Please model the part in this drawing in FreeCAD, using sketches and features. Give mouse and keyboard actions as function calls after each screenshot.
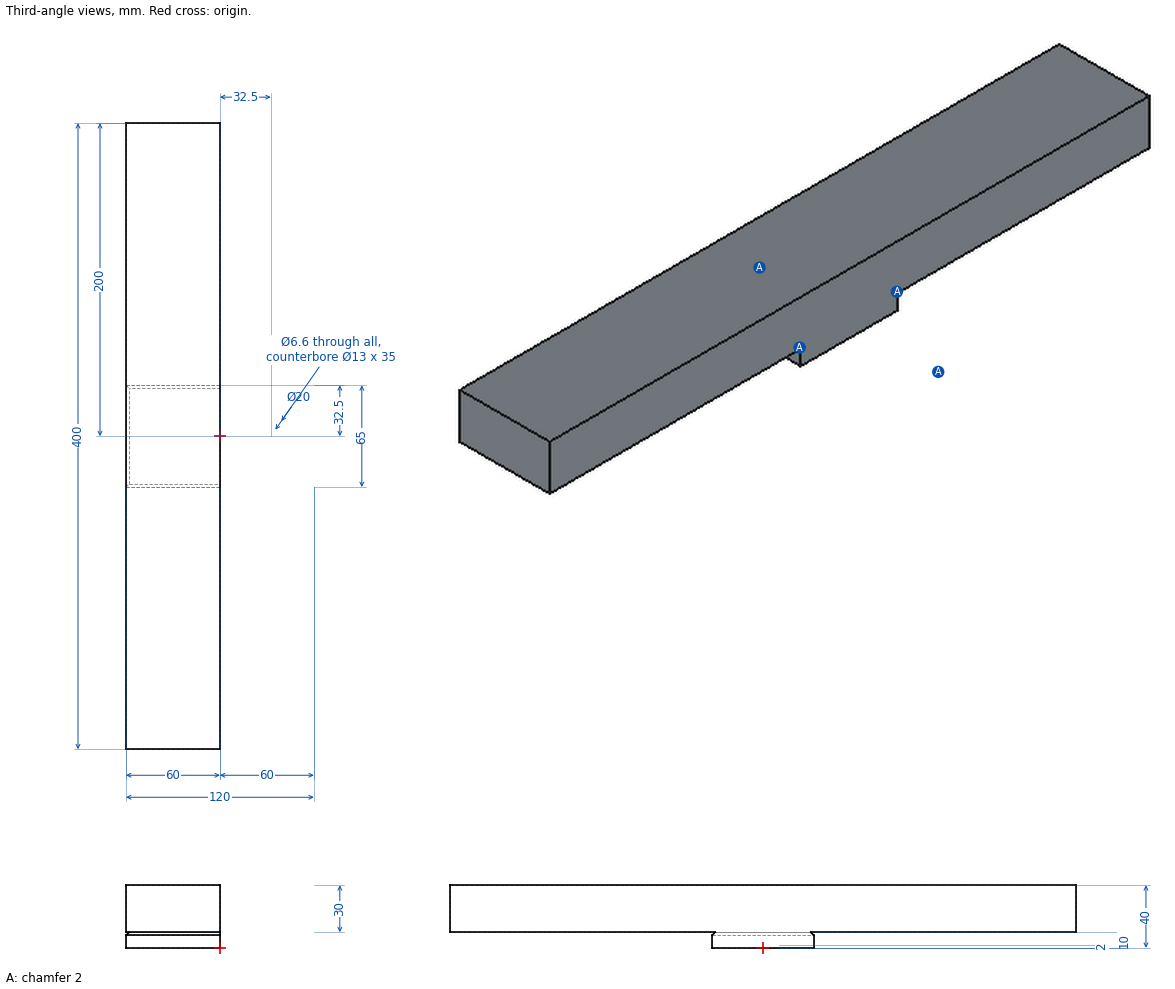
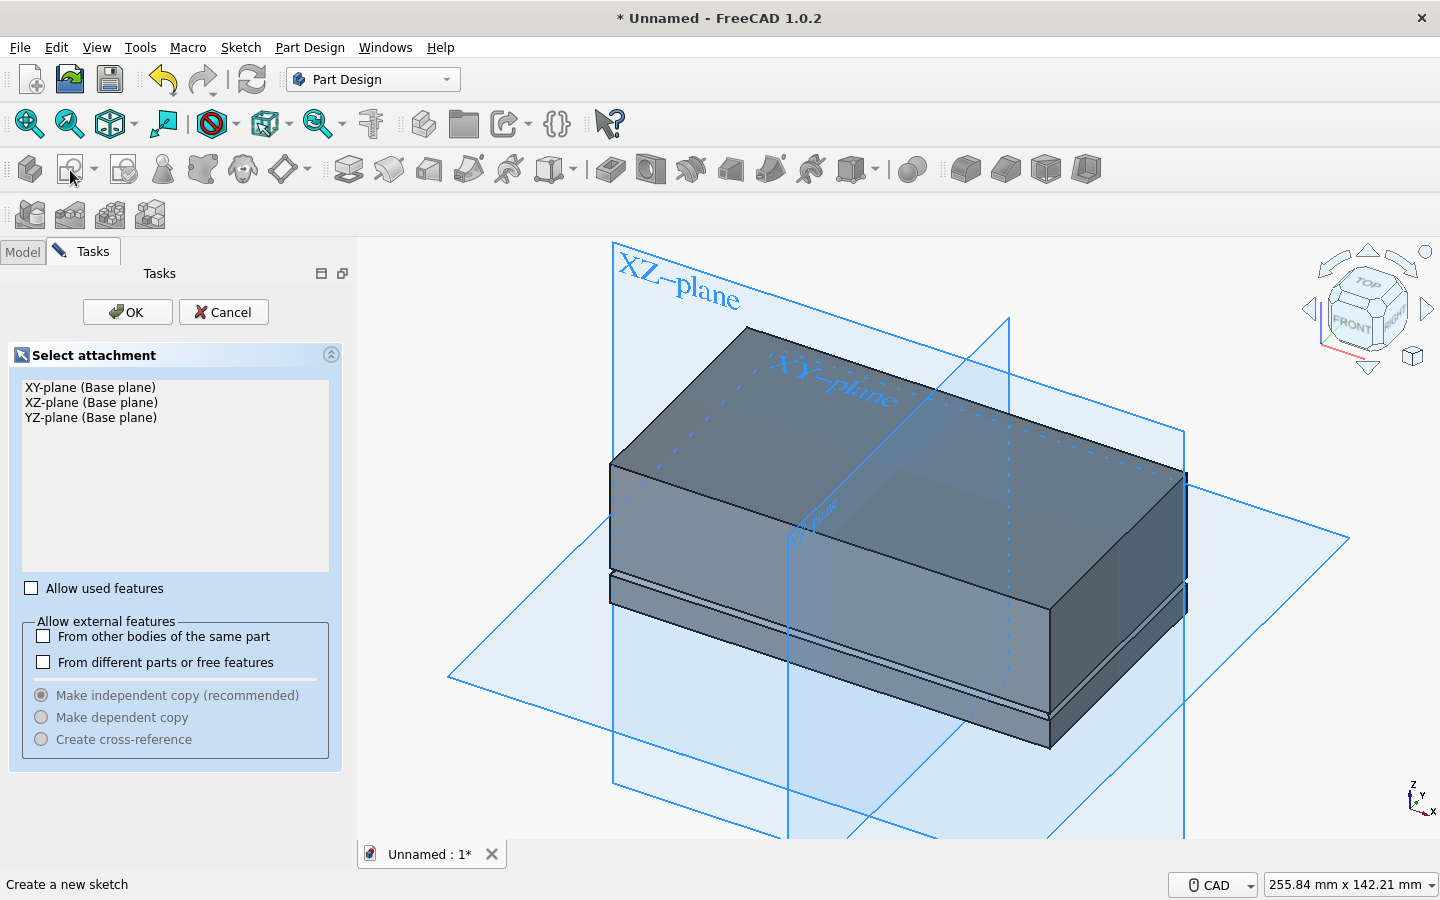
click(82, 388)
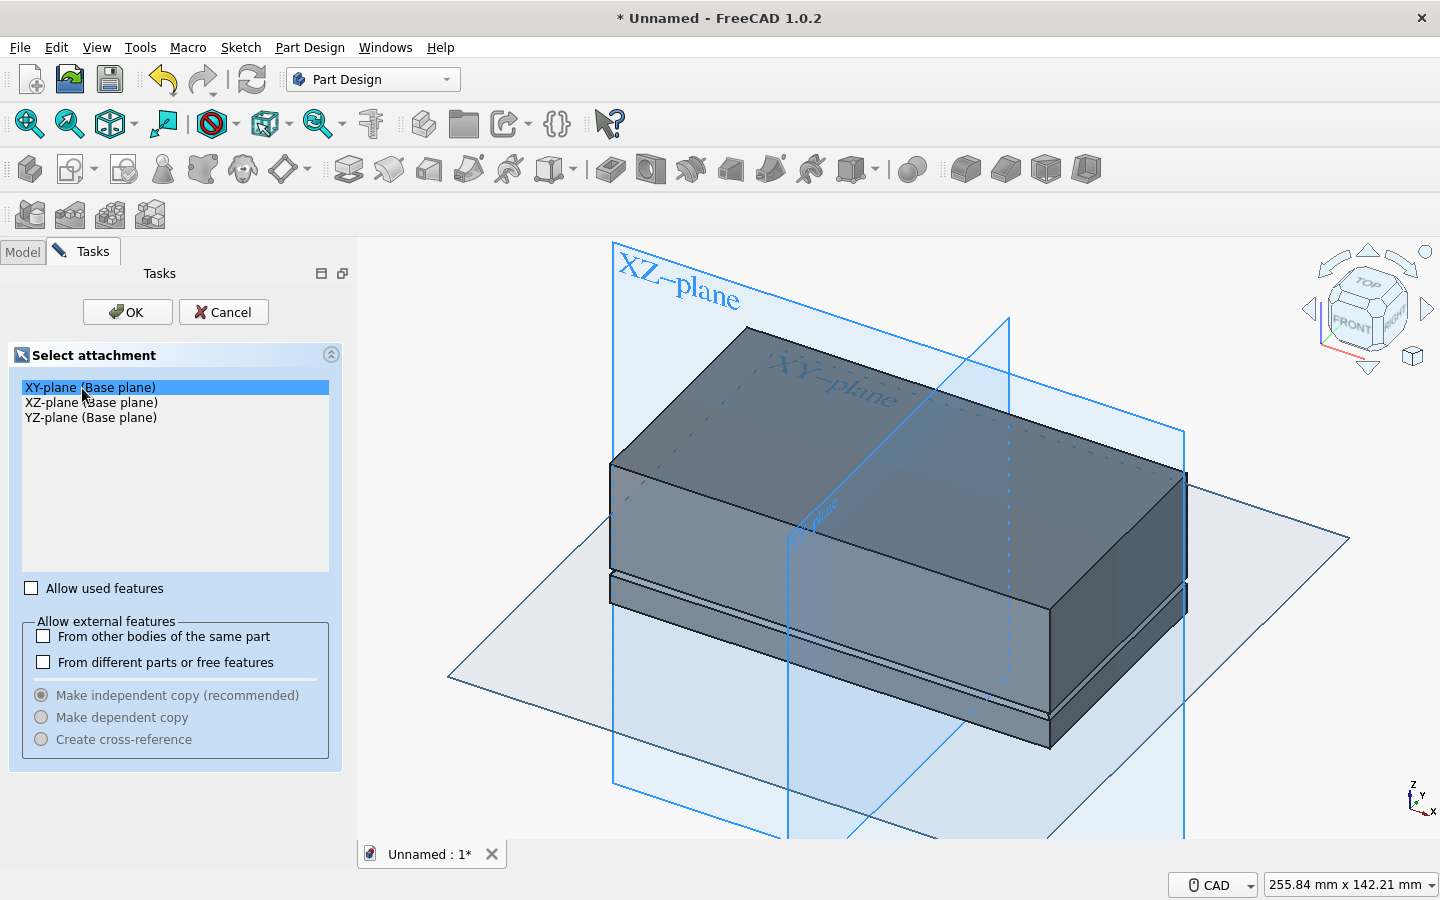
click(128, 312)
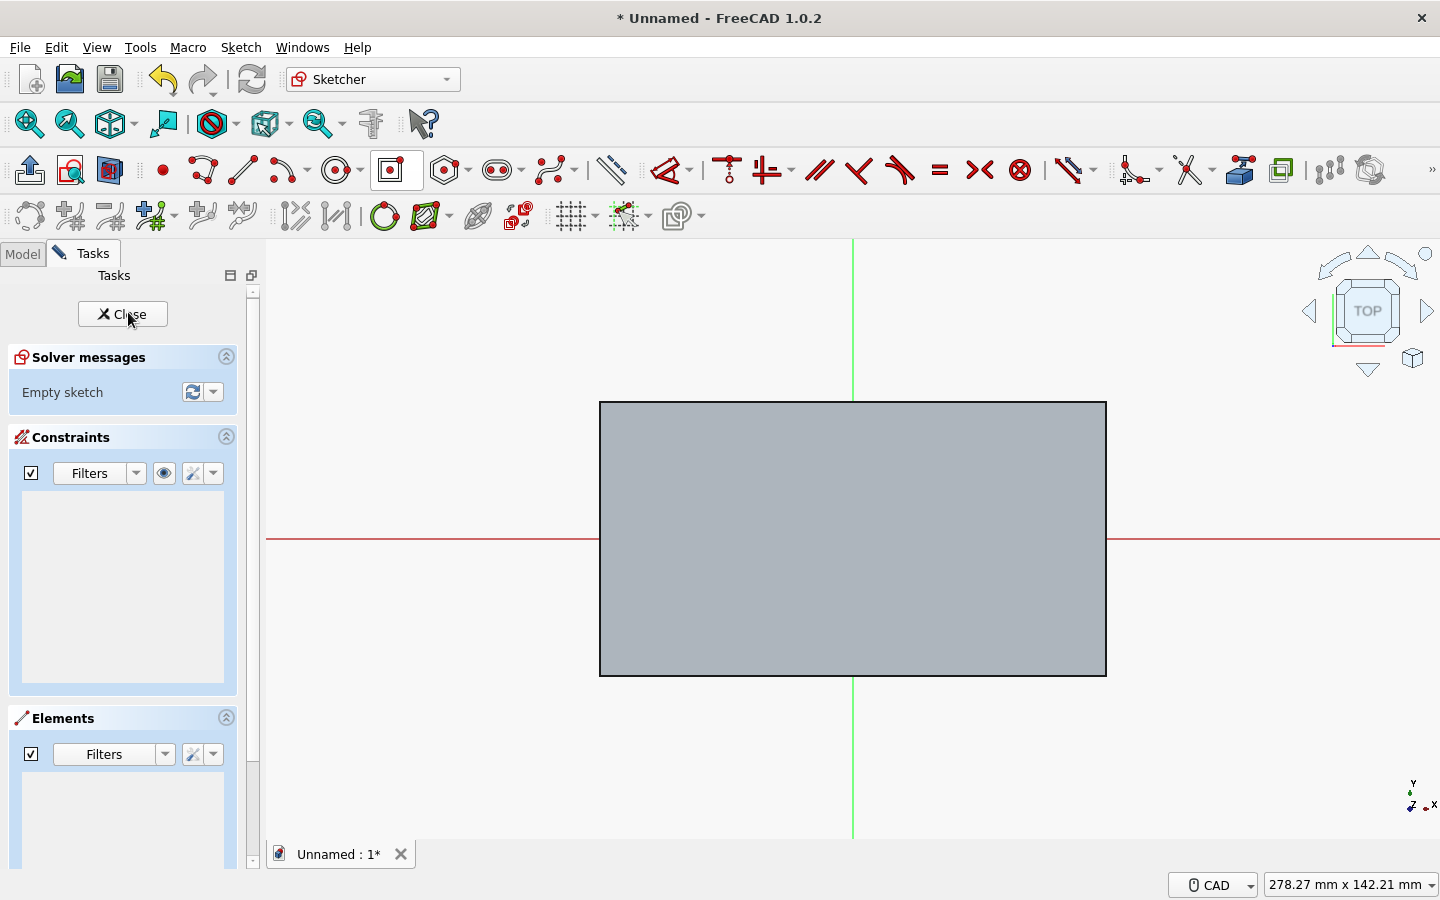
click(110, 170)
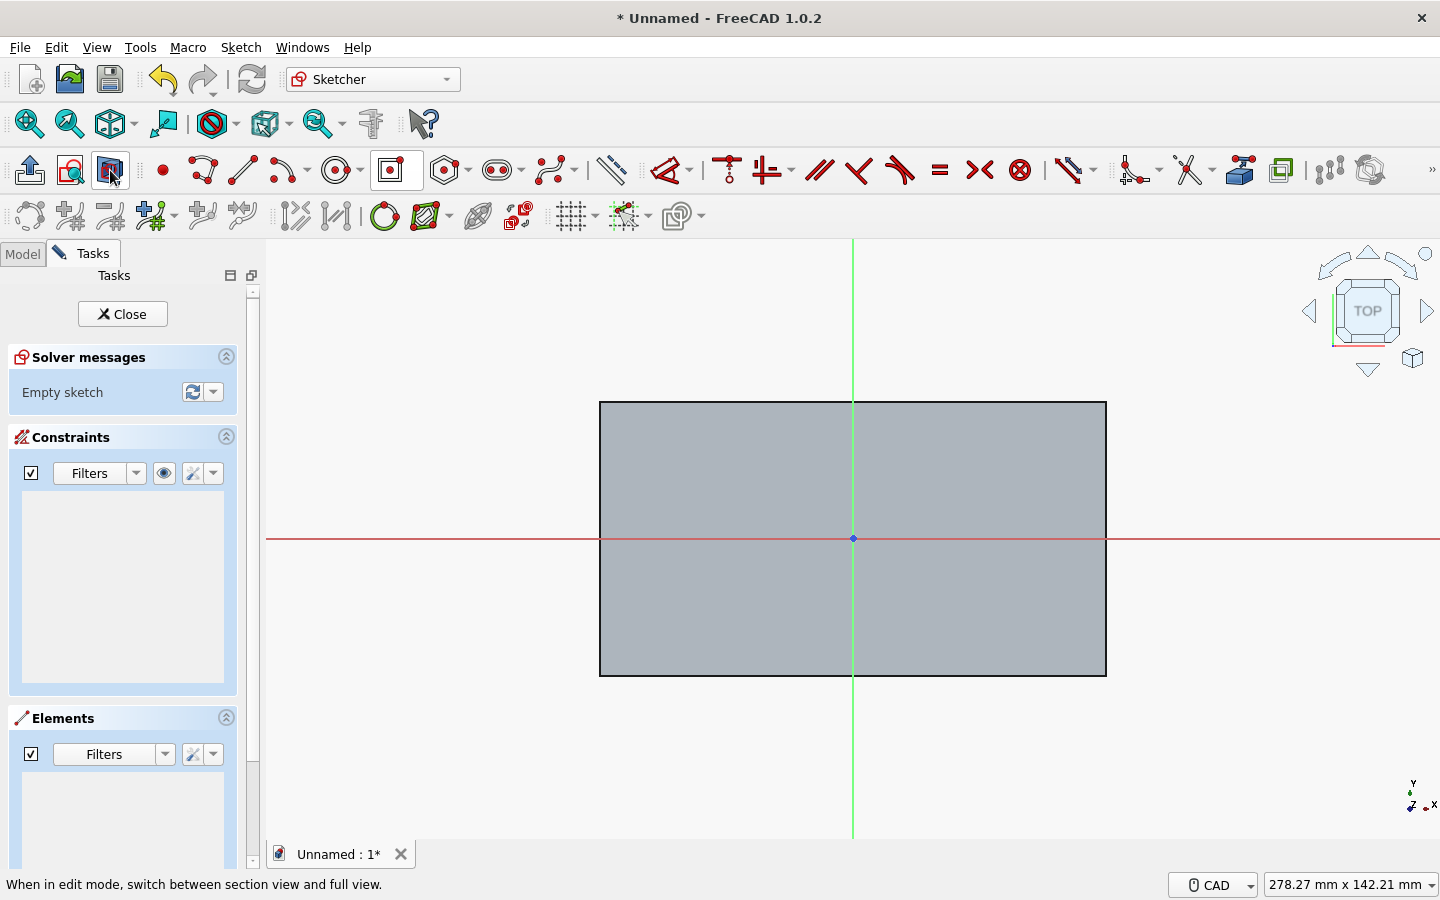
scroll(994, 539, up, 7)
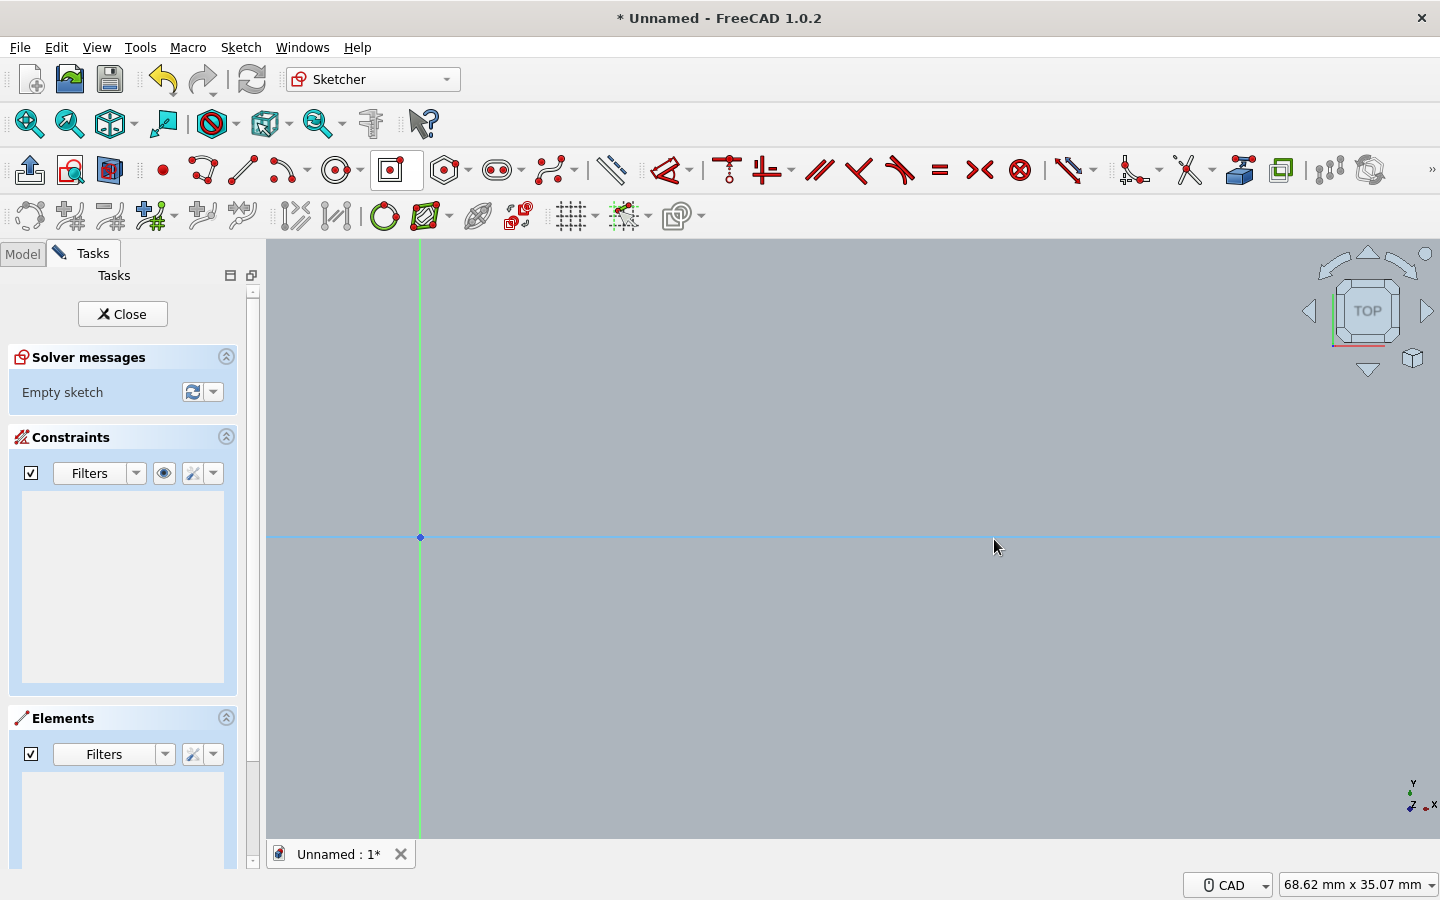
click(336, 170)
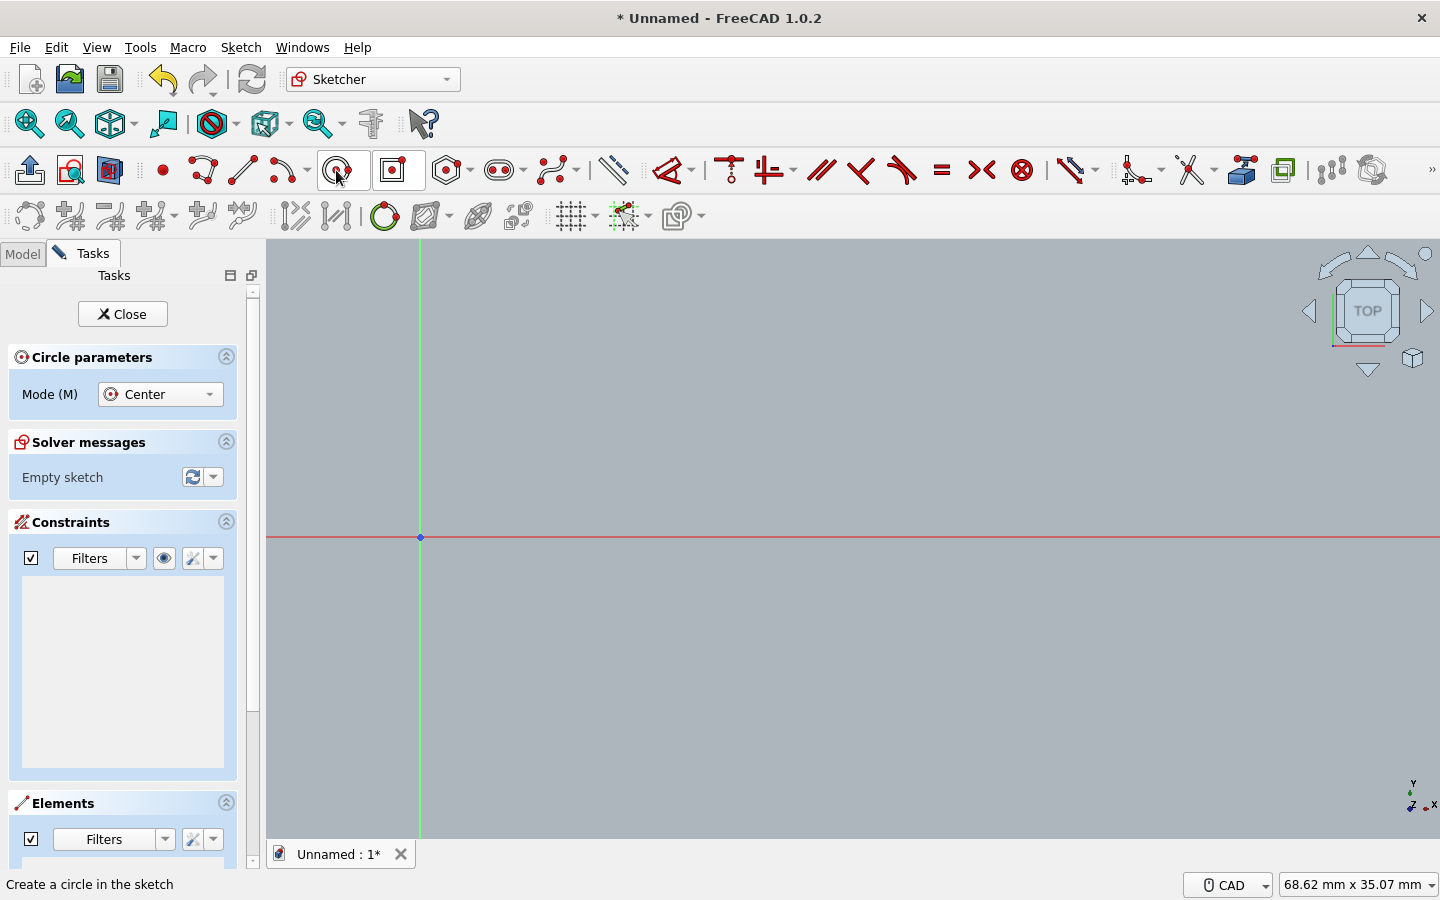
click(976, 537)
click(1097, 416)
key(Escape)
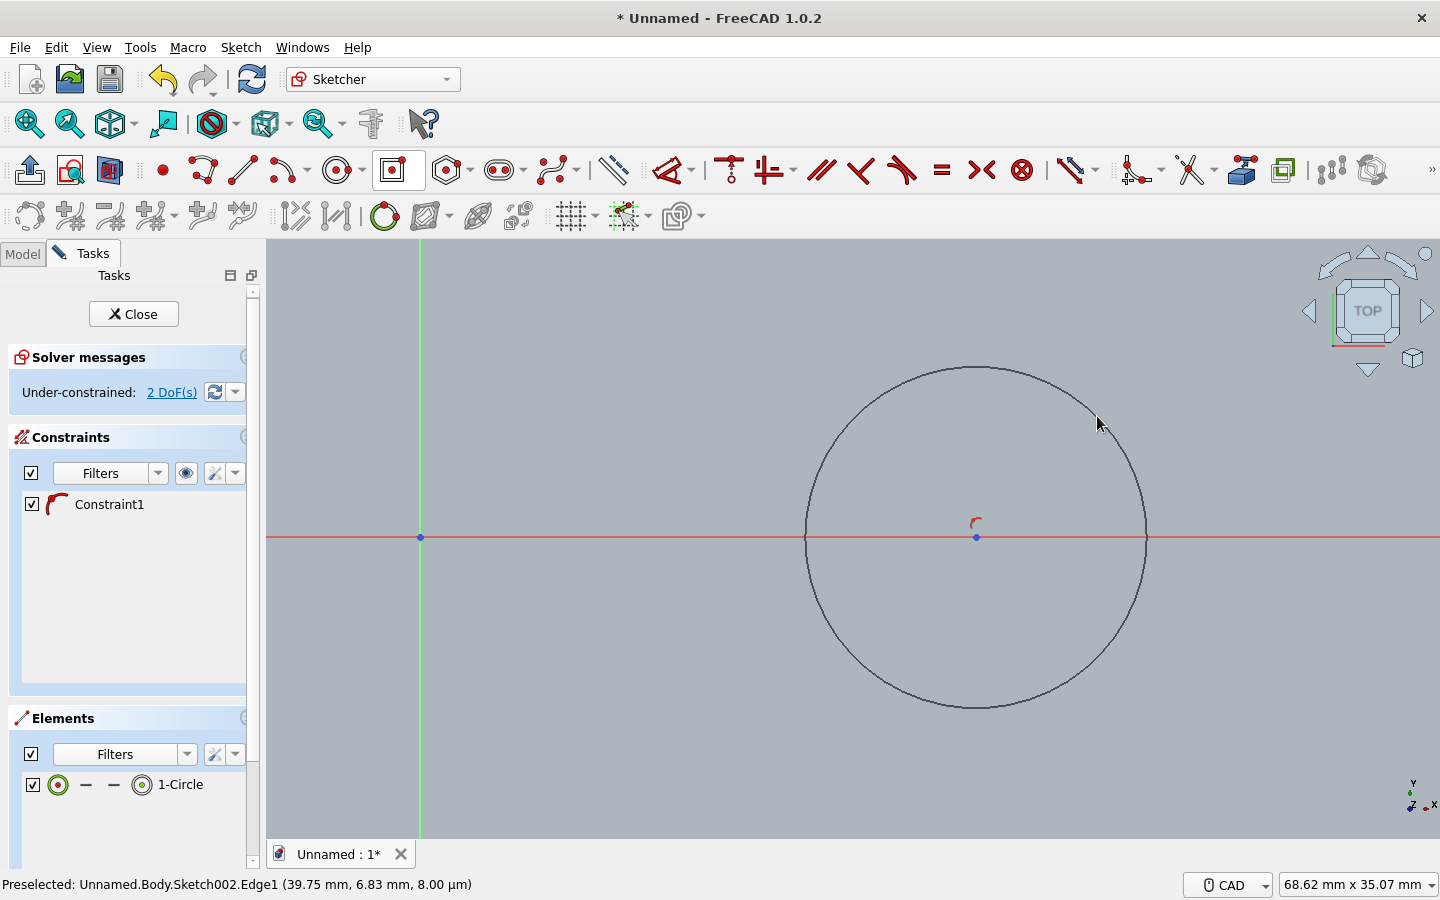
click(668, 170)